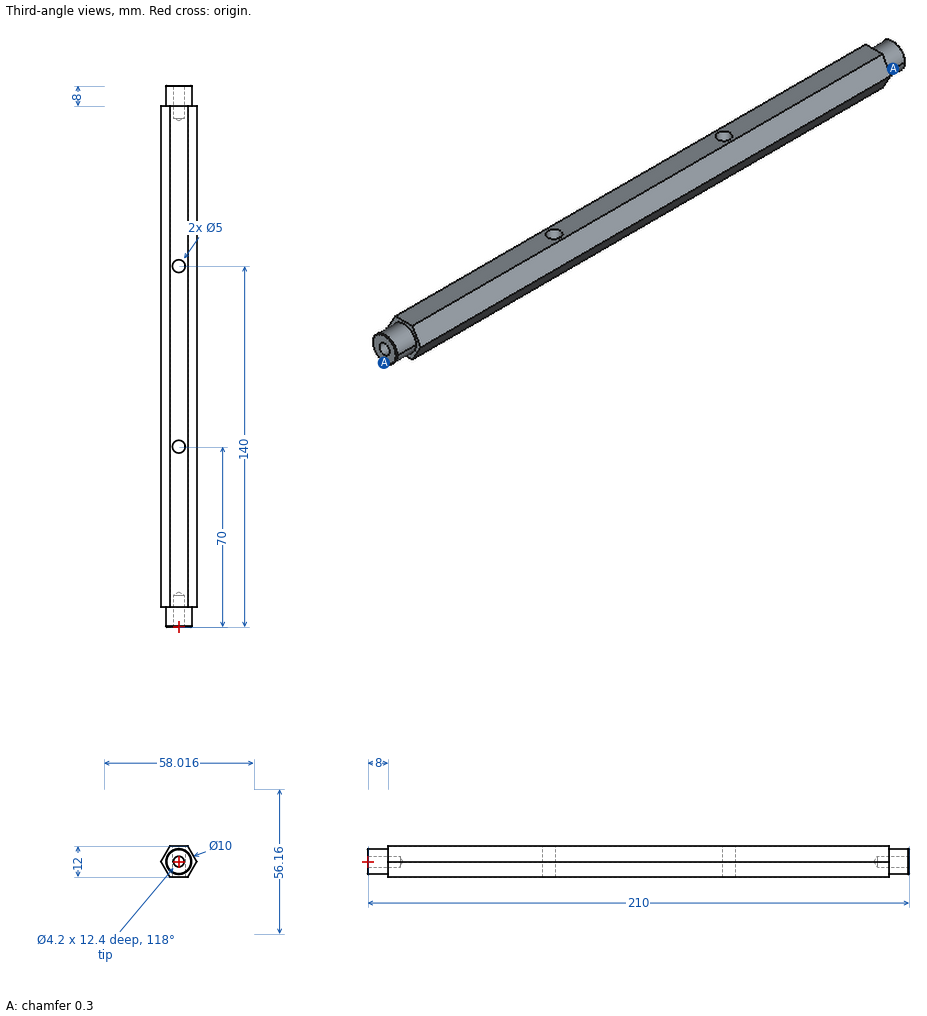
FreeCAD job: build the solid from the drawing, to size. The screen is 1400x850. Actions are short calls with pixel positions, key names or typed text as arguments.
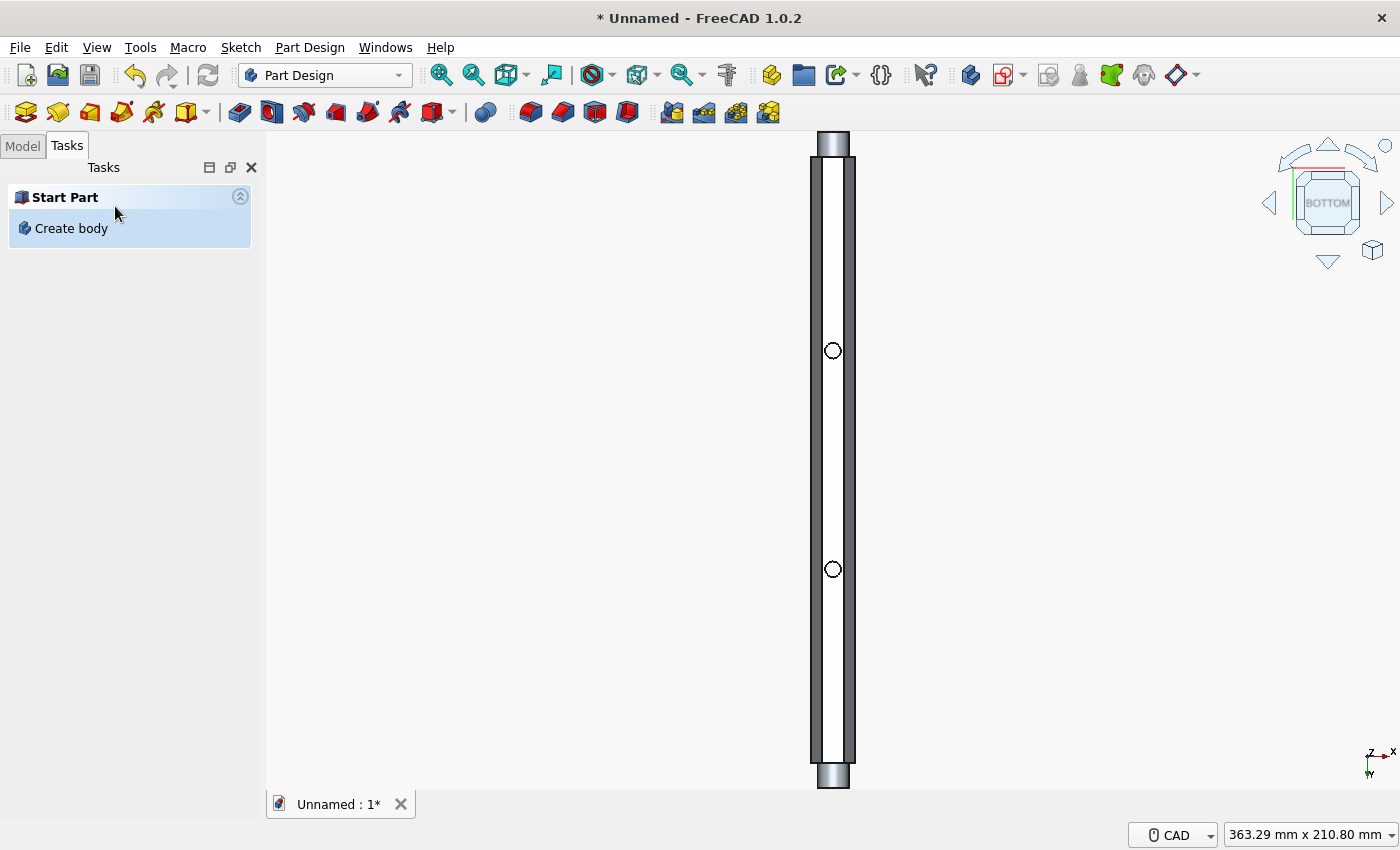
click(1004, 76)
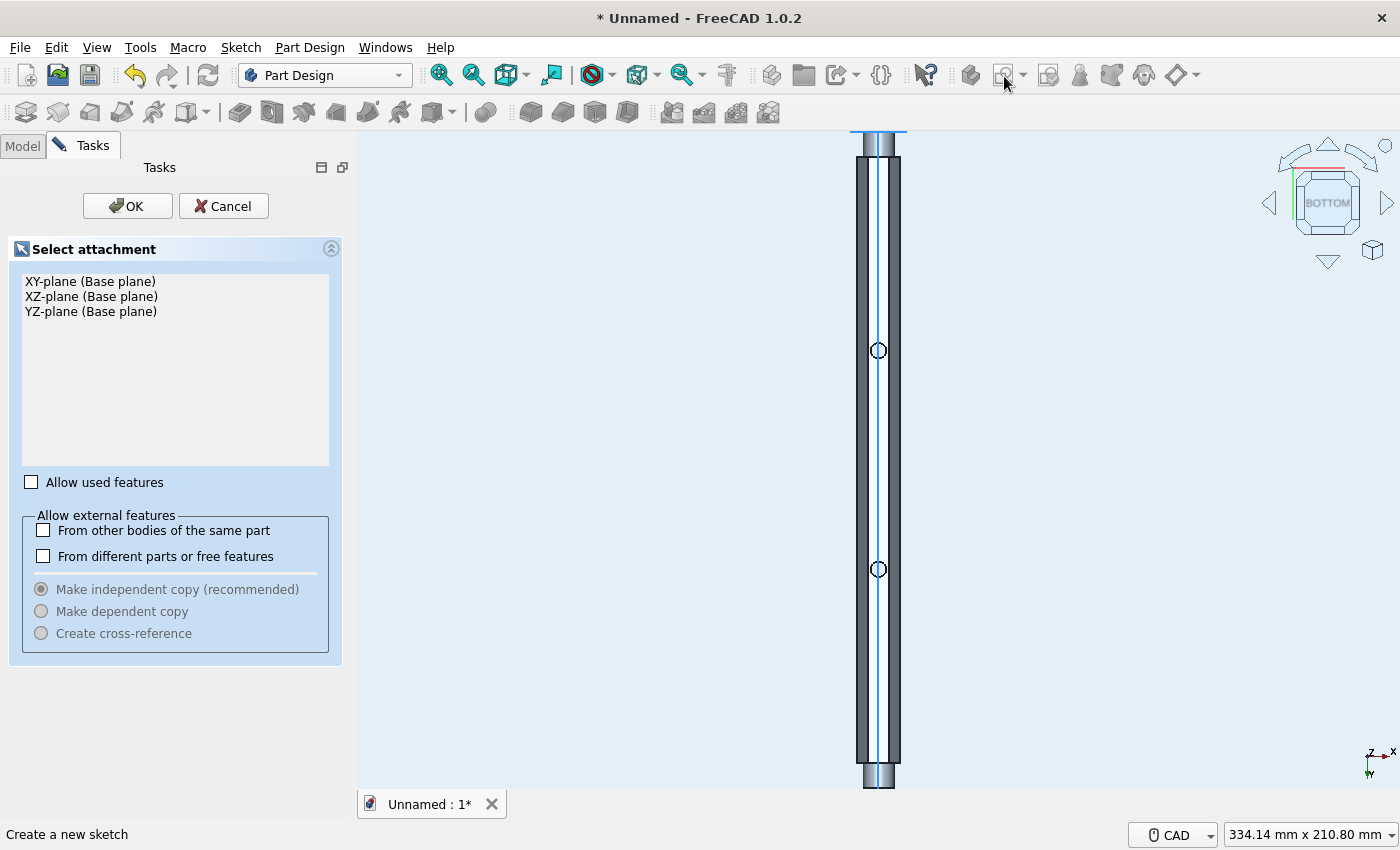
click(82, 296)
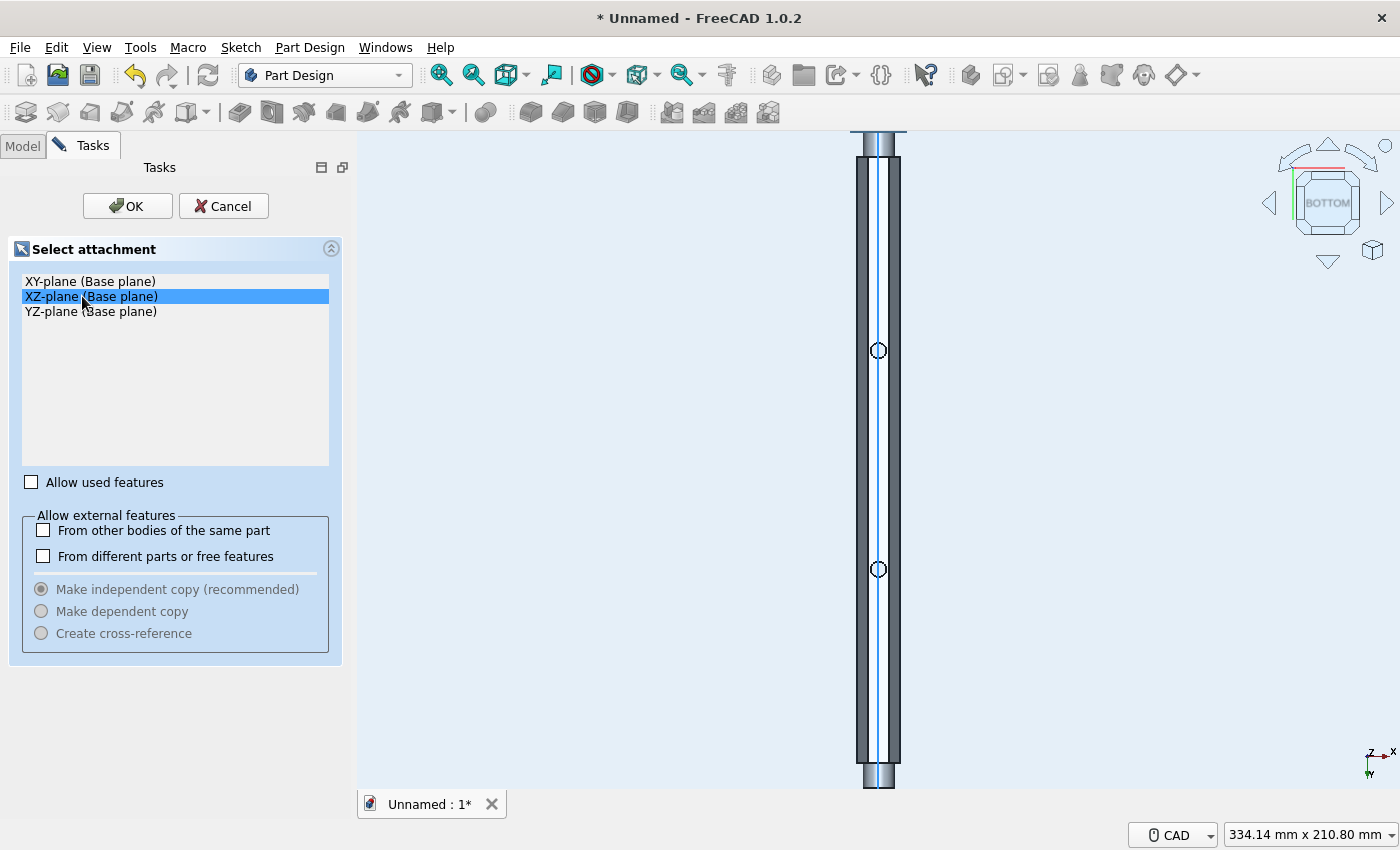
click(128, 206)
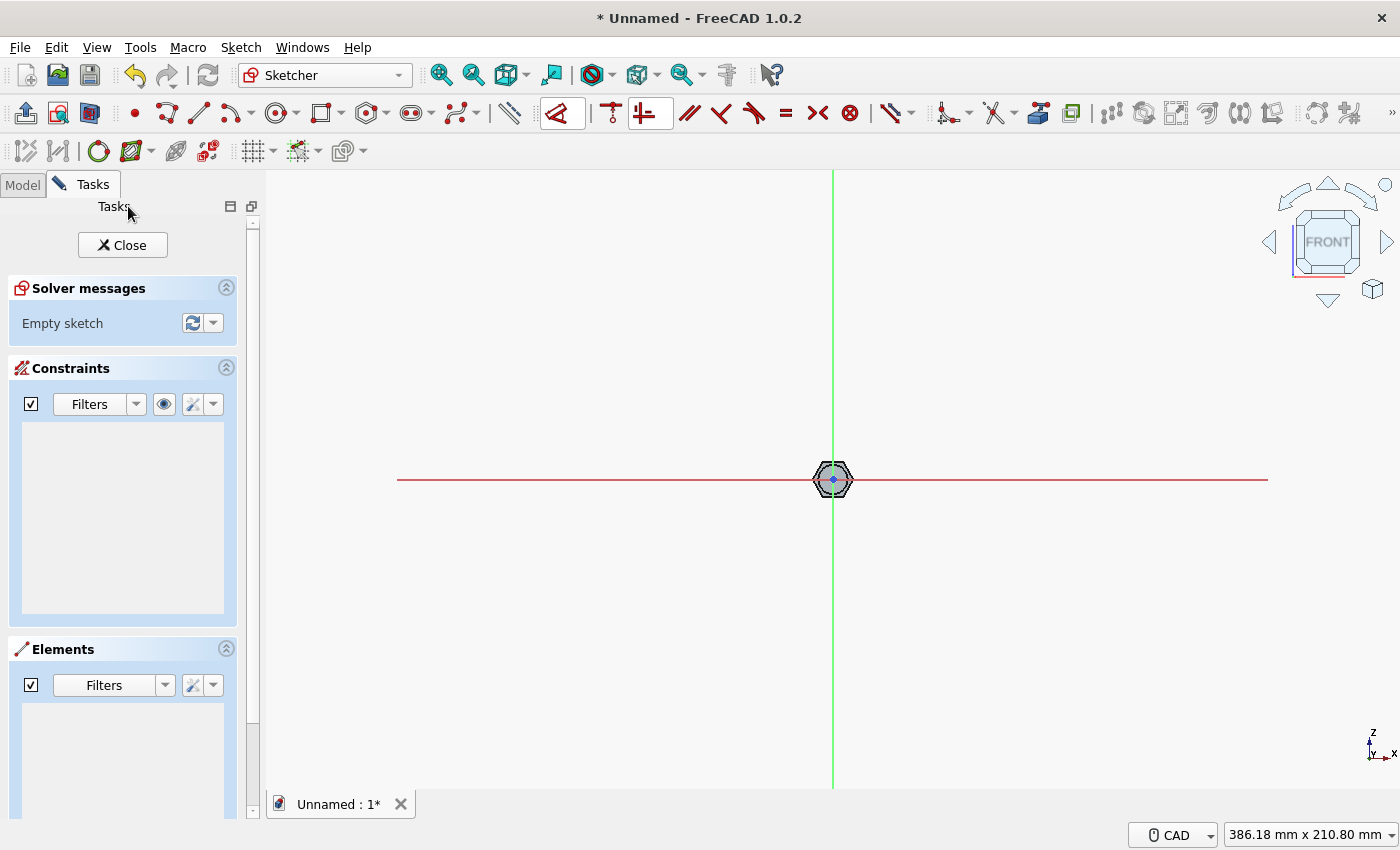
scroll(837, 480, up, 15)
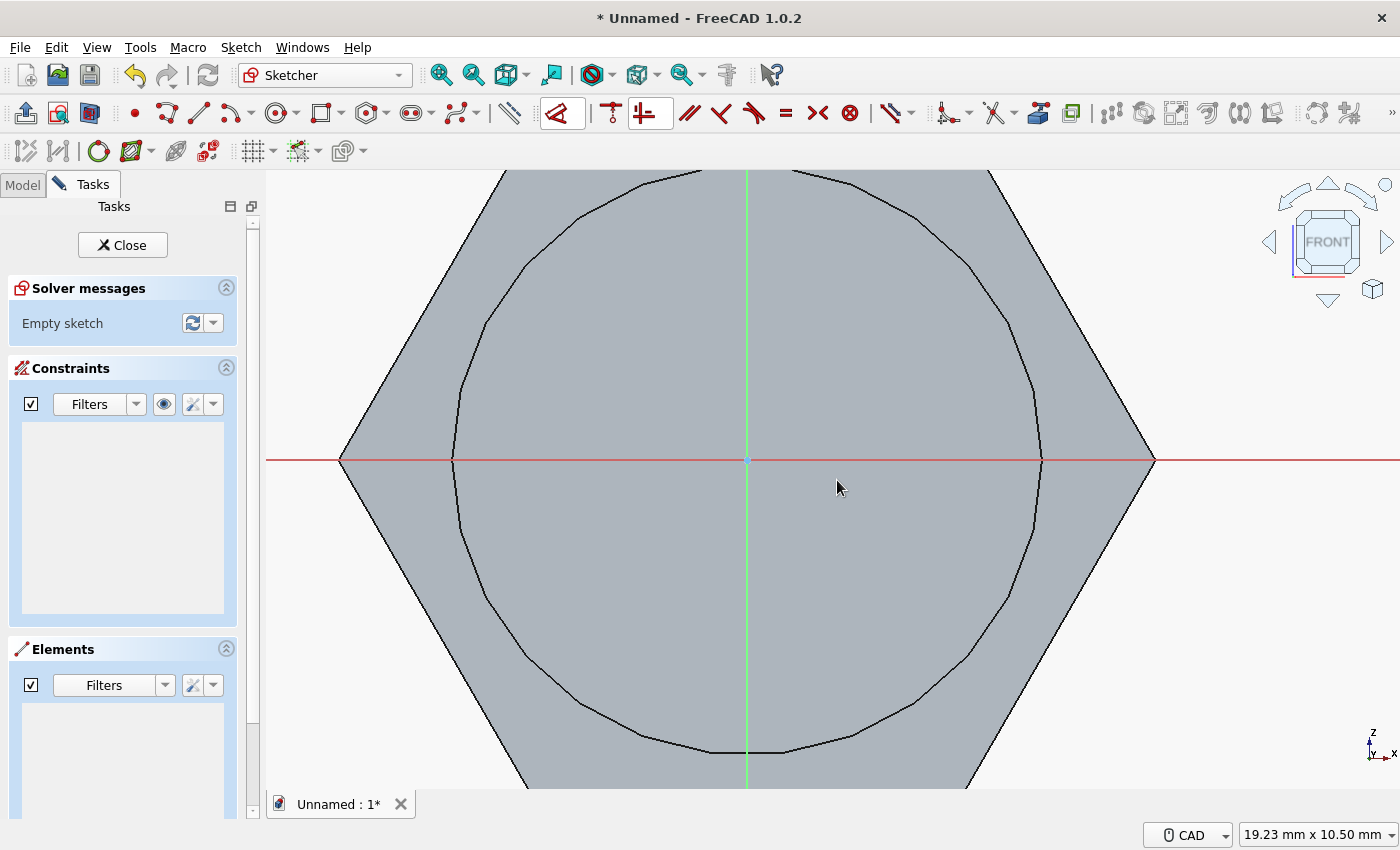
scroll(712, 422, up, 2)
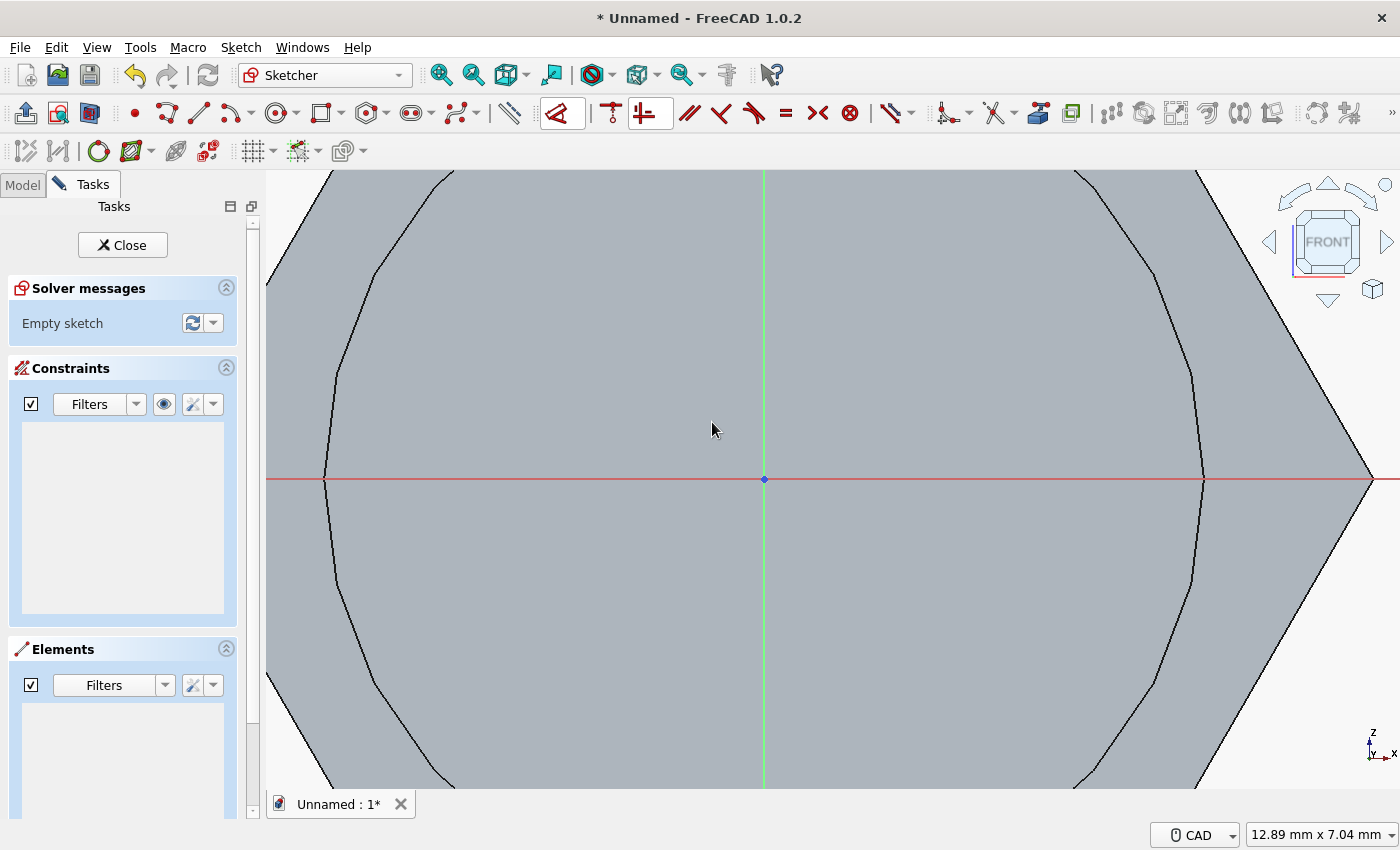
key(g)
key(c)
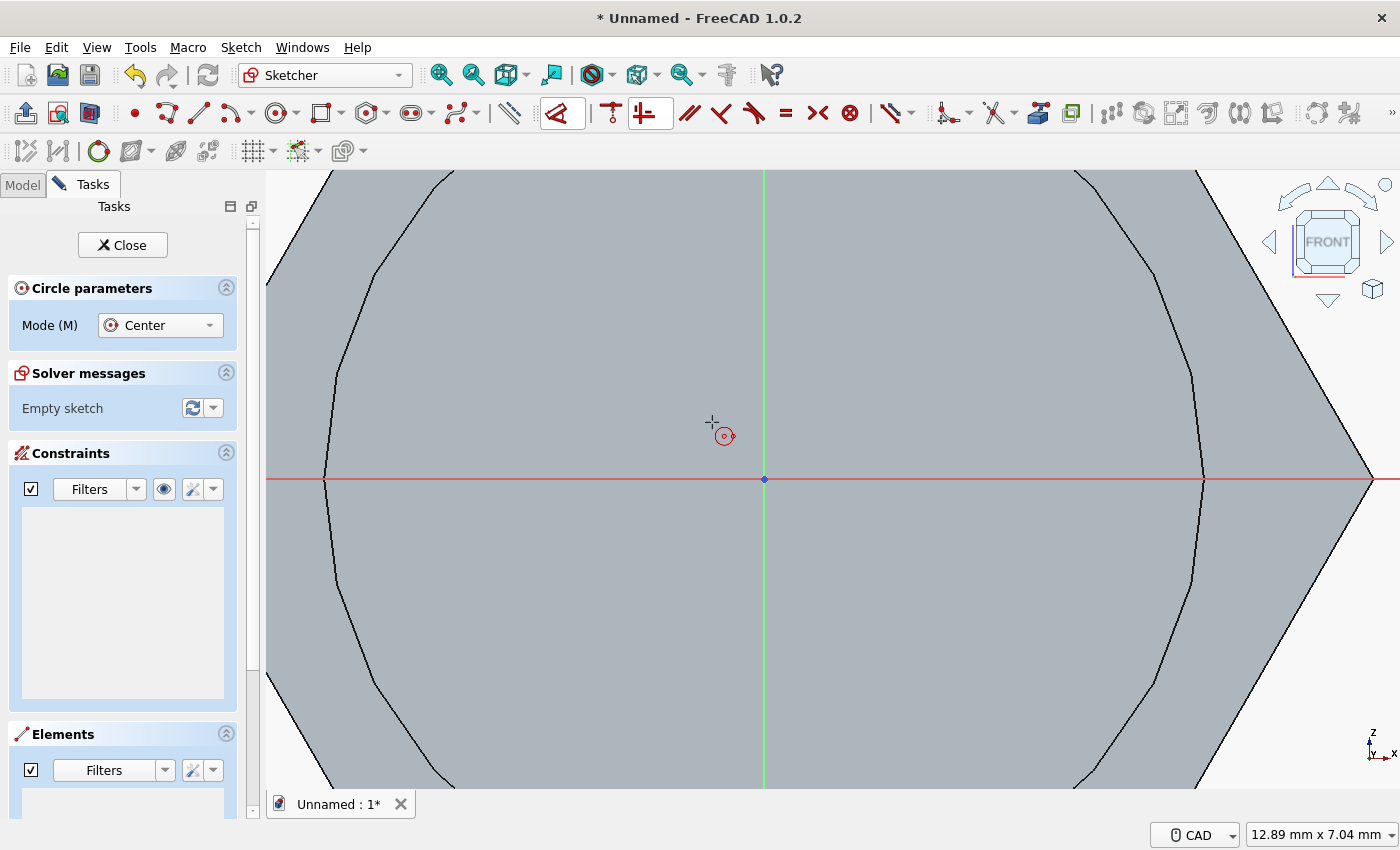
click(764, 479)
click(895, 348)
key(Escape)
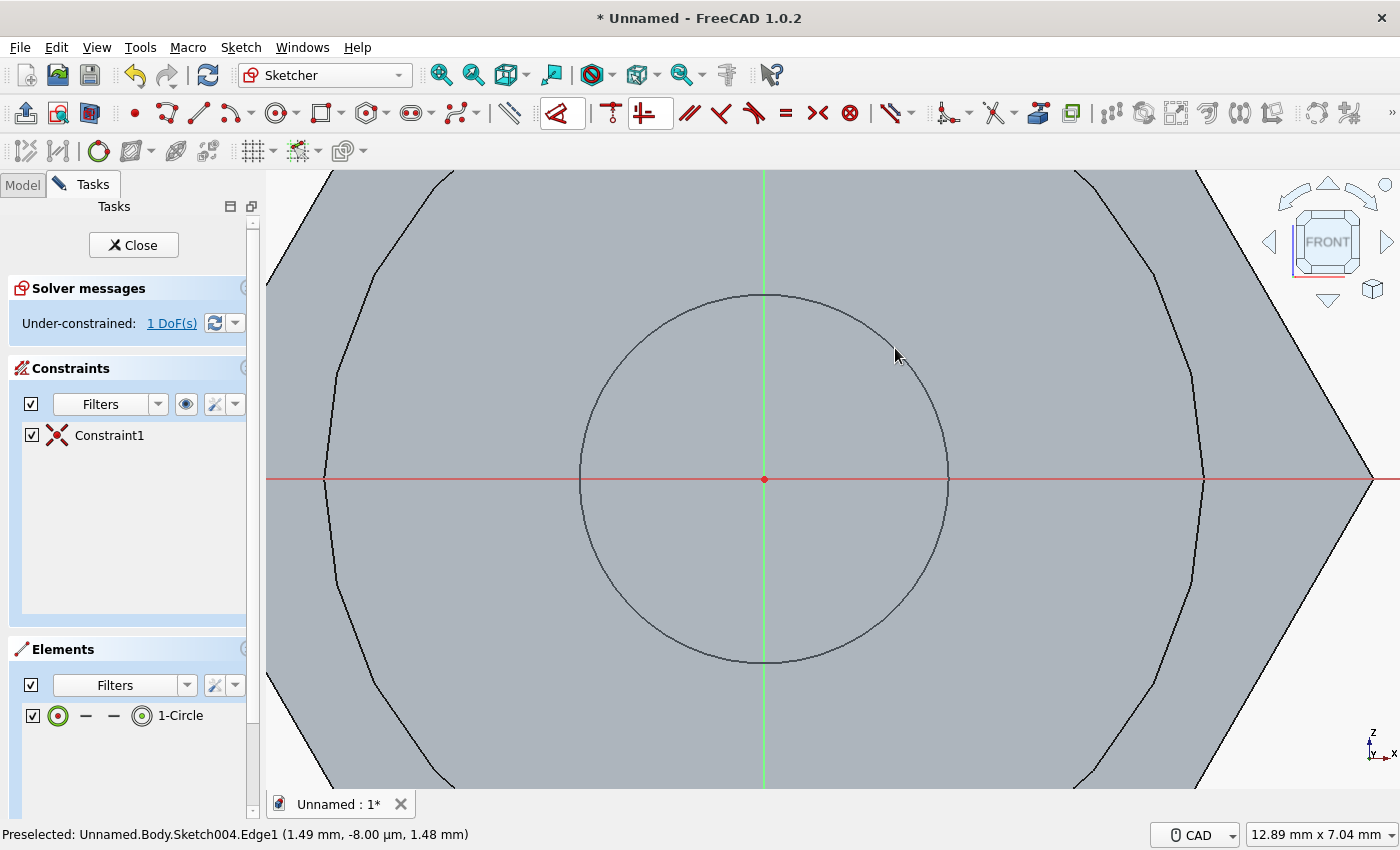
click(894, 348)